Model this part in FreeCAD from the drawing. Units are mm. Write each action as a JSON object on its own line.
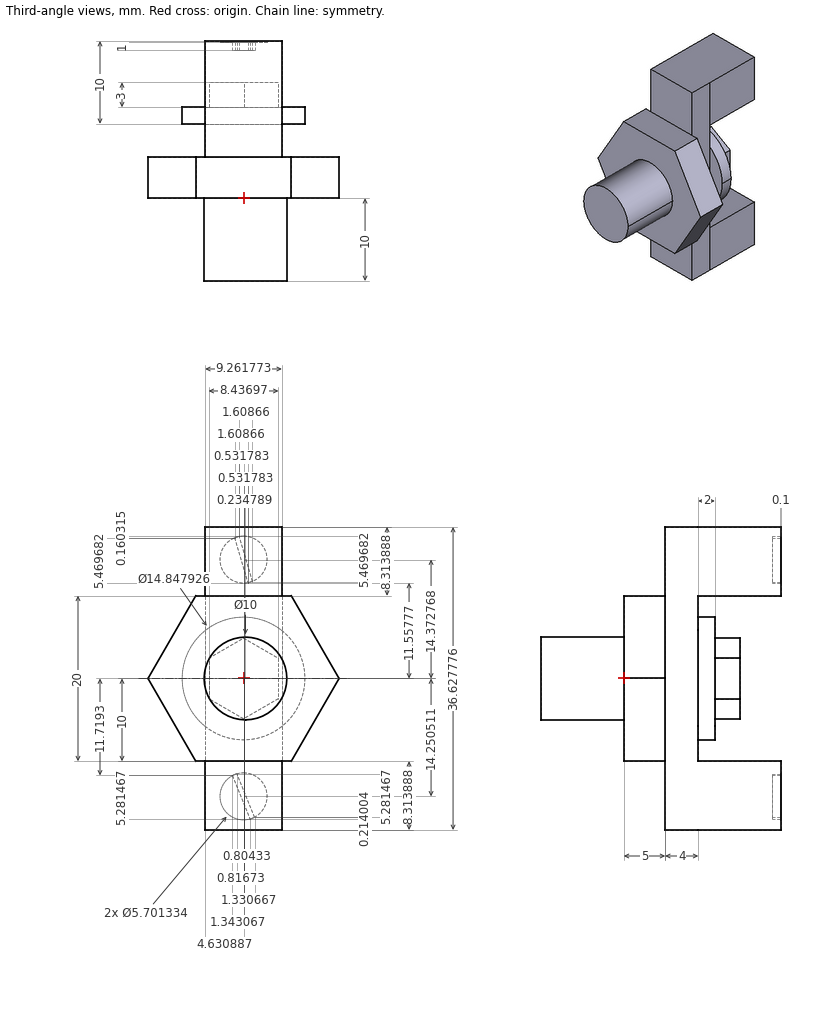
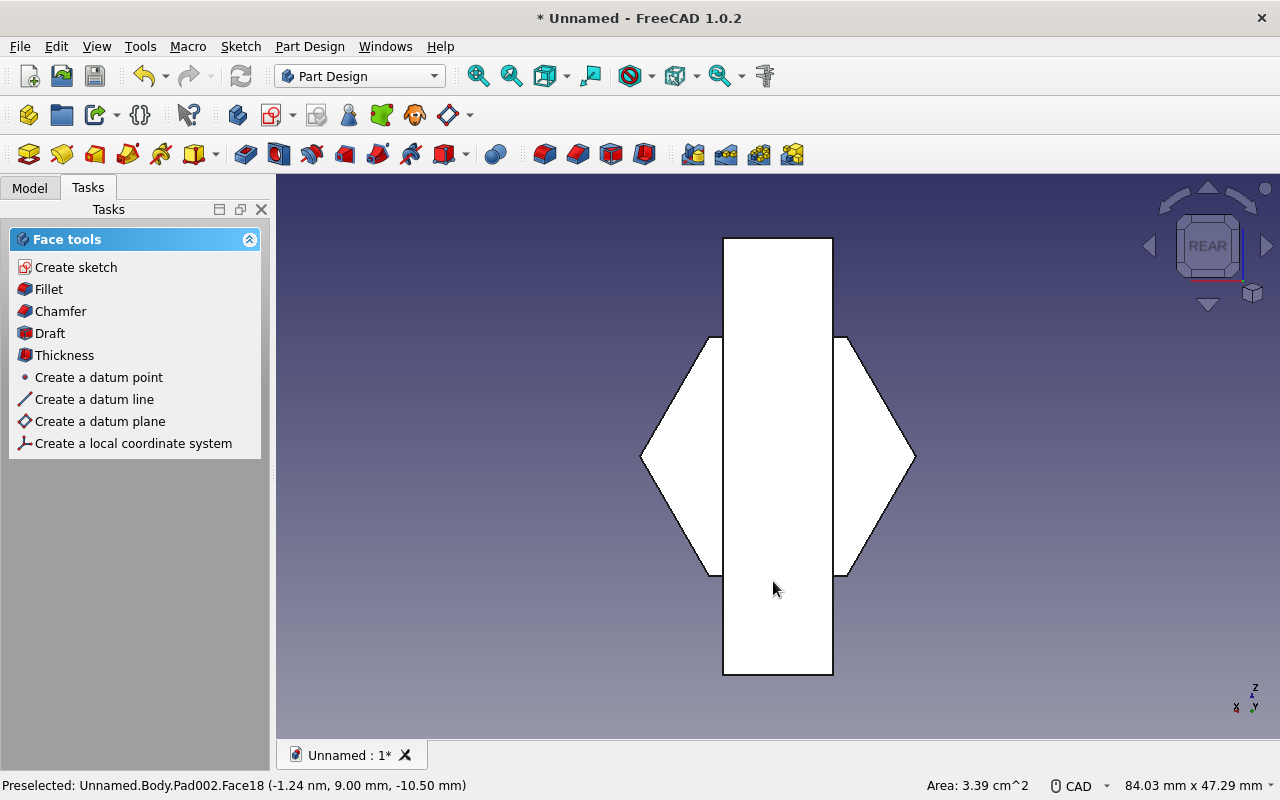
{"action": "left_click", "coordinate": [270, 116]}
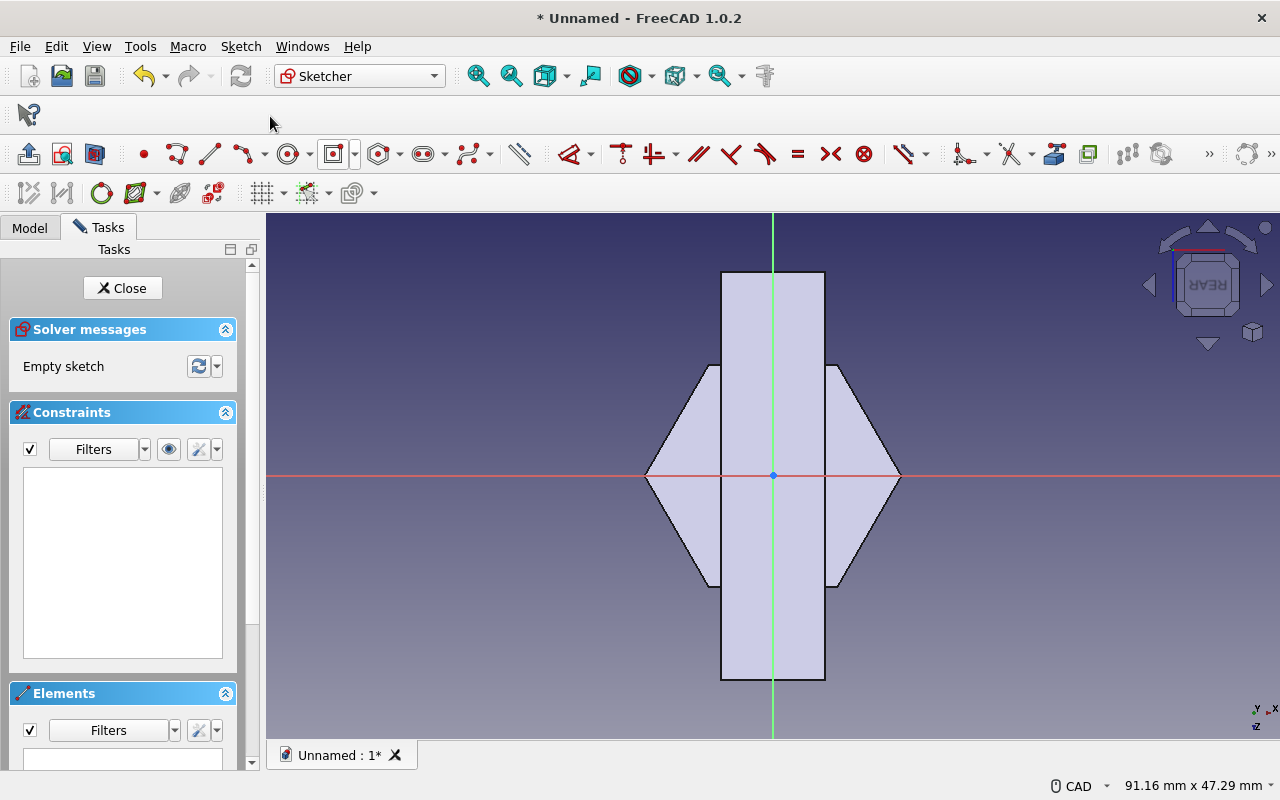
{"action": "left_click", "coordinate": [354, 154]}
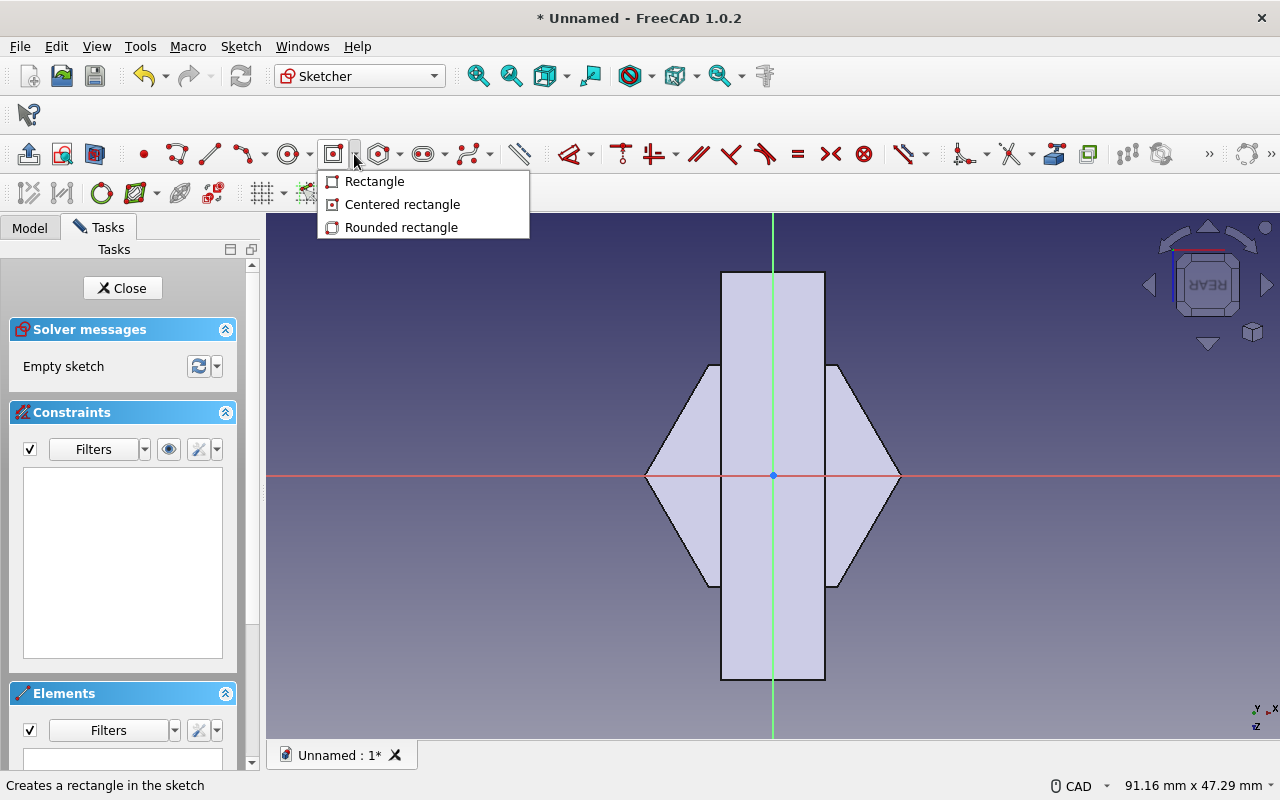
{"action": "left_click", "coordinate": [424, 182]}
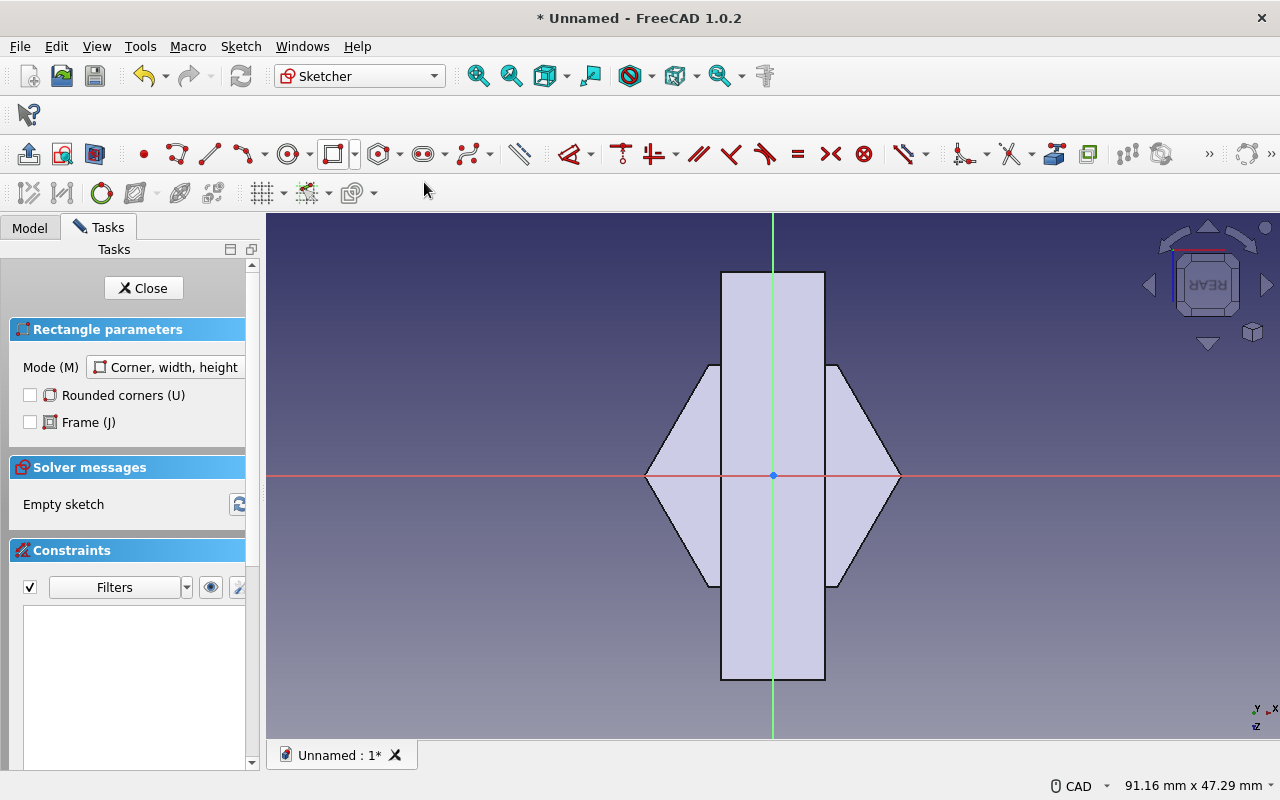
{"action": "left_click", "coordinate": [721, 272]}
{"action": "mouse_move", "coordinate": [825, 365]}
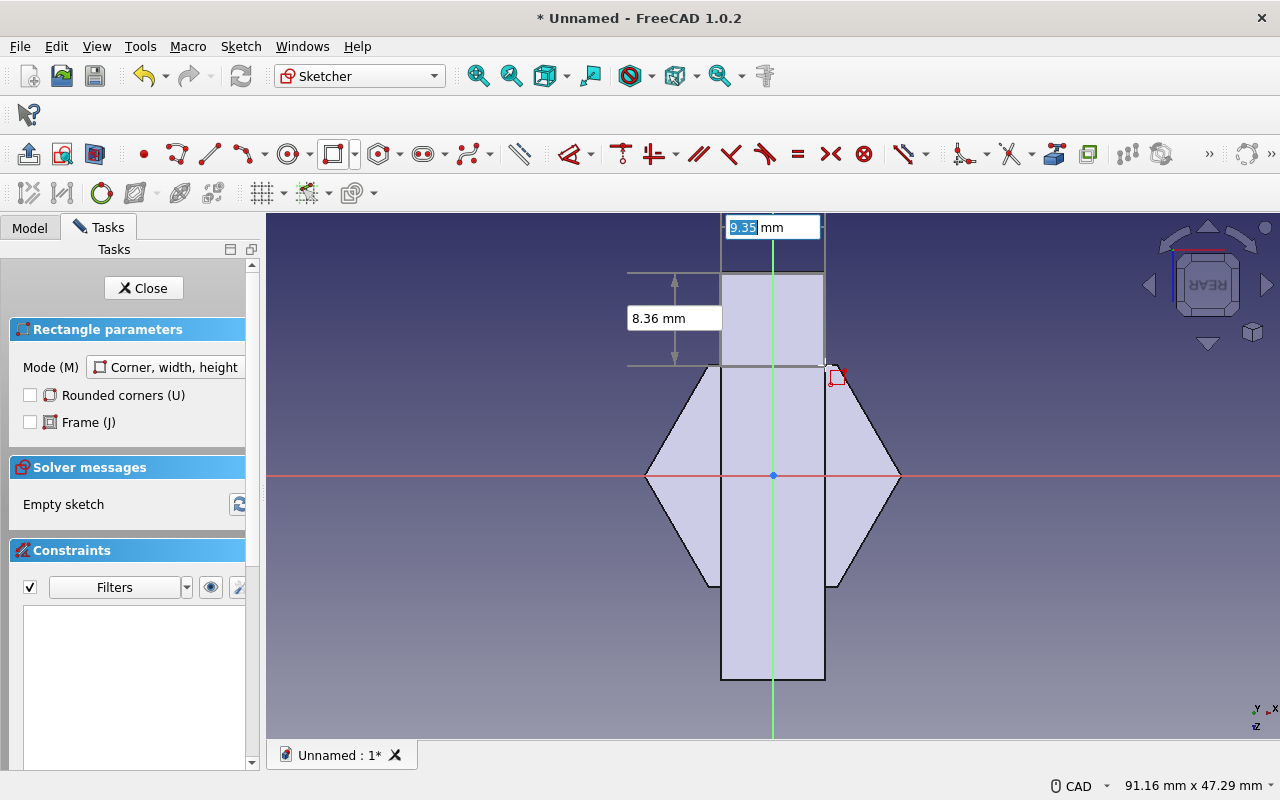
{"action": "type", "text": "9.261773"}
{"action": "key", "text": "Tab"}
{"action": "type", "text": "8.313888"}
{"action": "key", "text": "Return"}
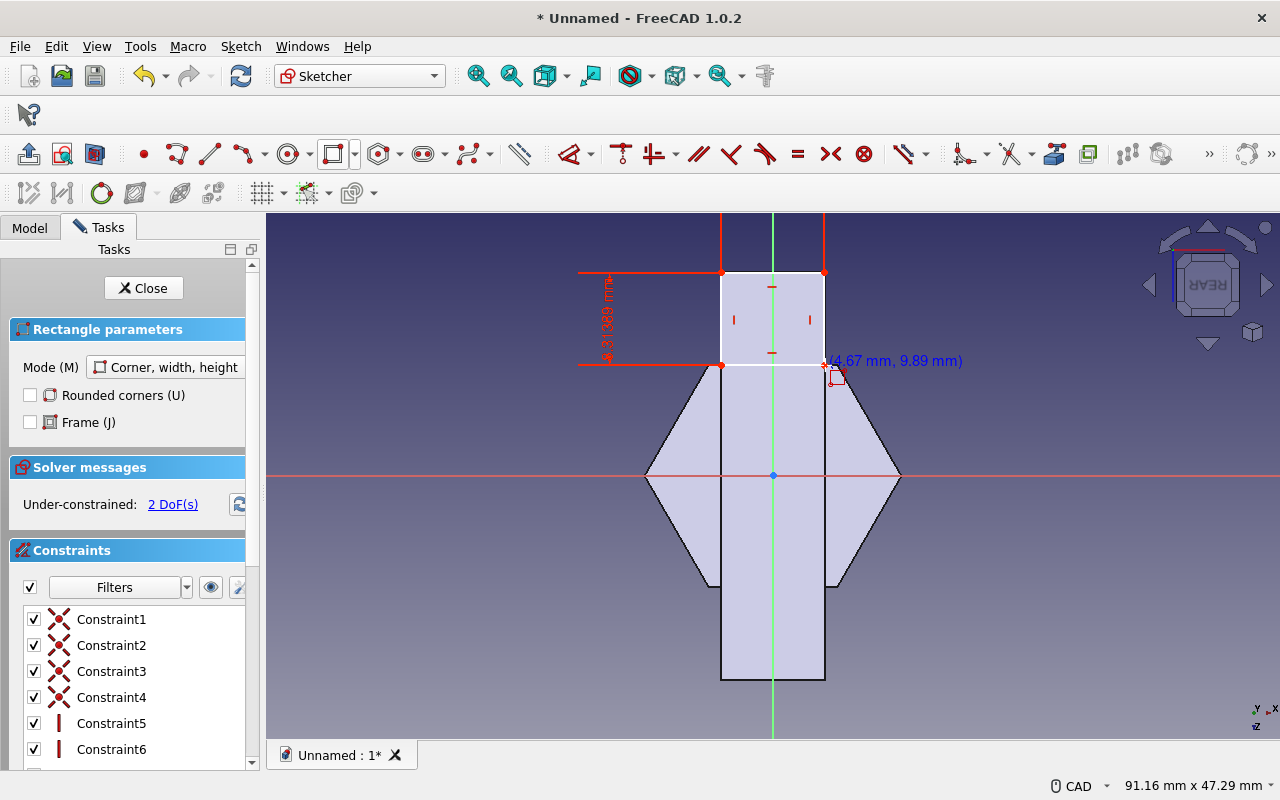
{"action": "left_click", "coordinate": [721, 587]}
{"action": "mouse_move", "coordinate": [825, 680]}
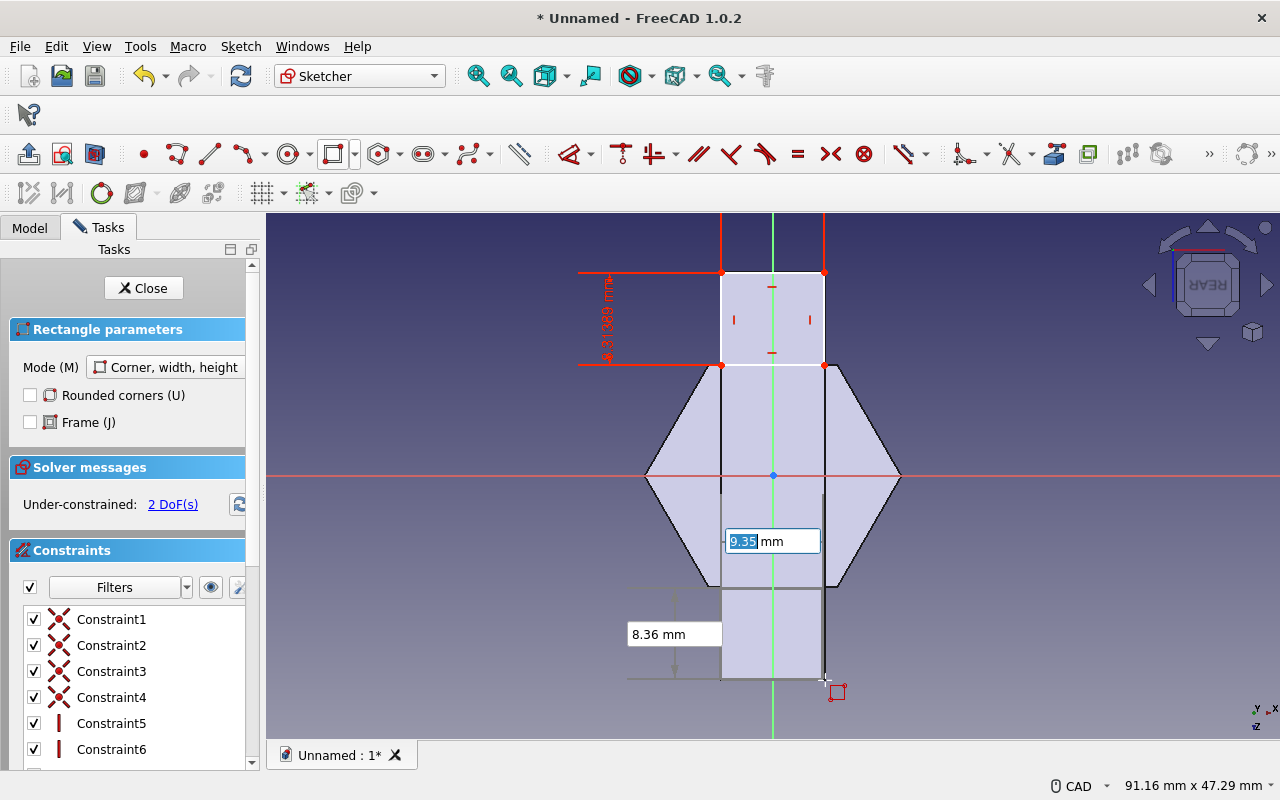
{"action": "type", "text": "9.261773"}
{"action": "key", "text": "Tab"}
{"action": "type", "text": "8.313888"}
{"action": "key", "text": "Return"}
{"action": "key", "text": "Escape"}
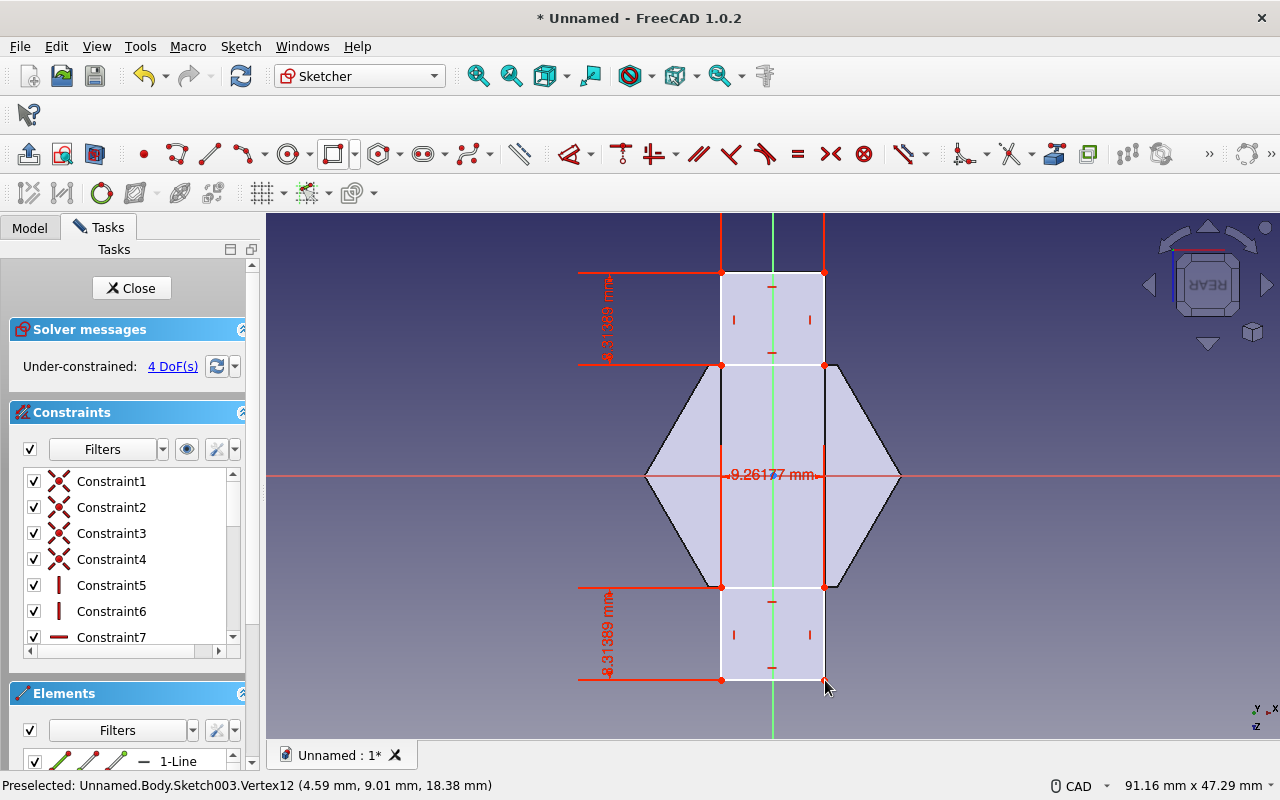
{"action": "left_click", "coordinate": [721, 365]}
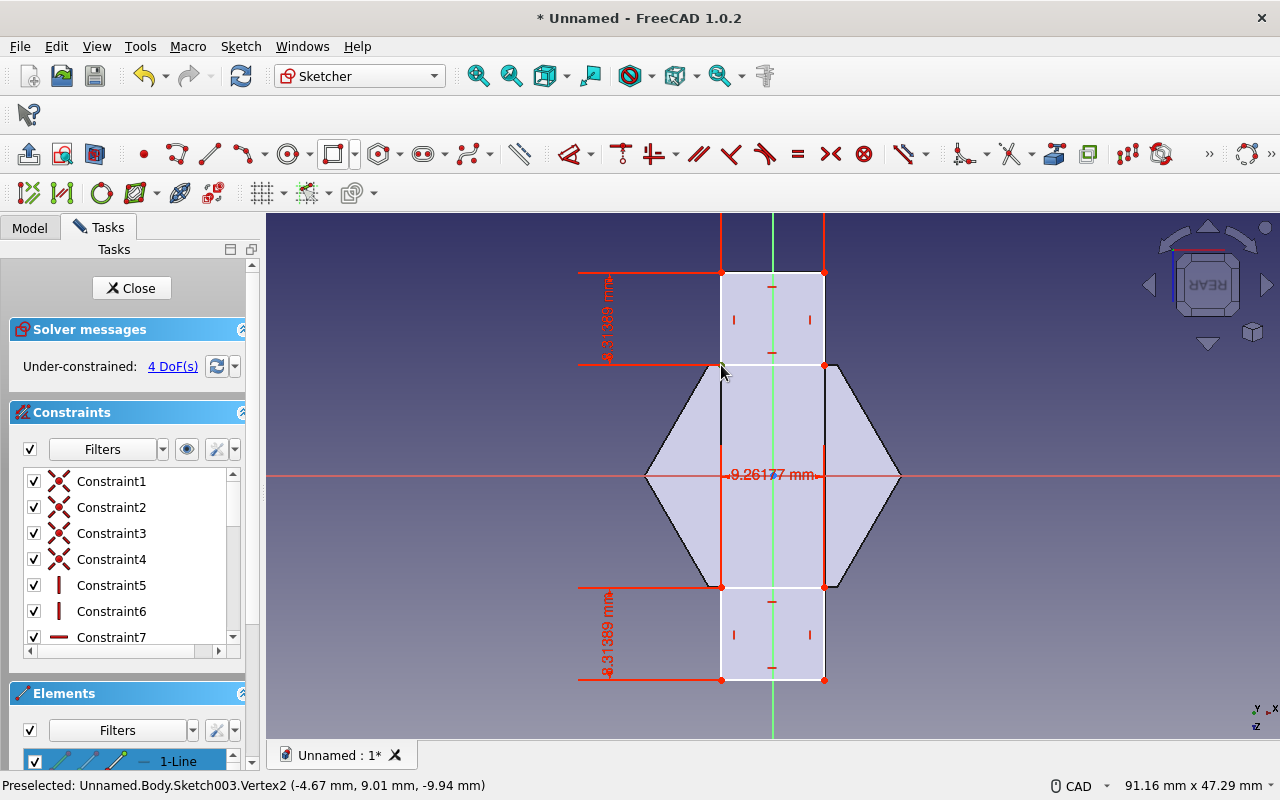
{"action": "left_click", "coordinate": [721, 588]}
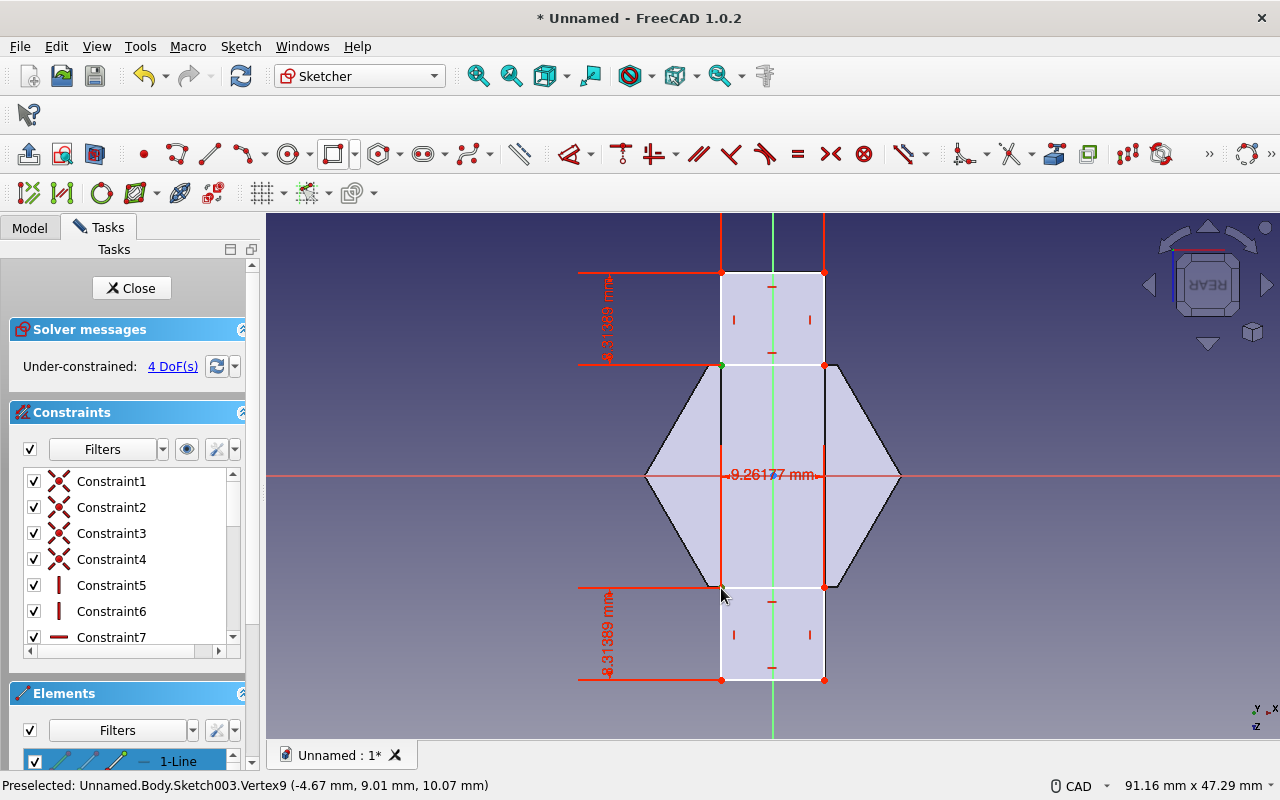
{"action": "left_click", "coordinate": [353, 476]}